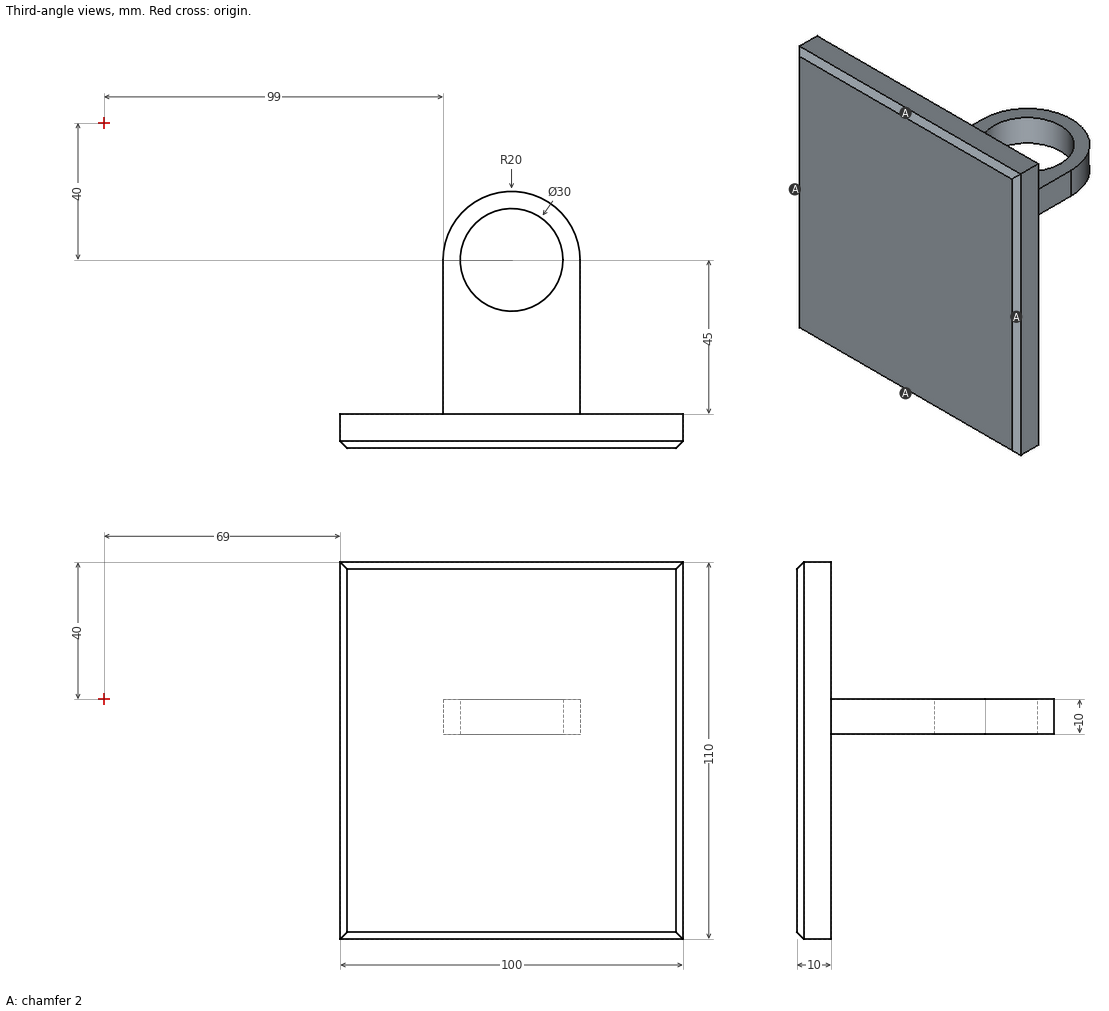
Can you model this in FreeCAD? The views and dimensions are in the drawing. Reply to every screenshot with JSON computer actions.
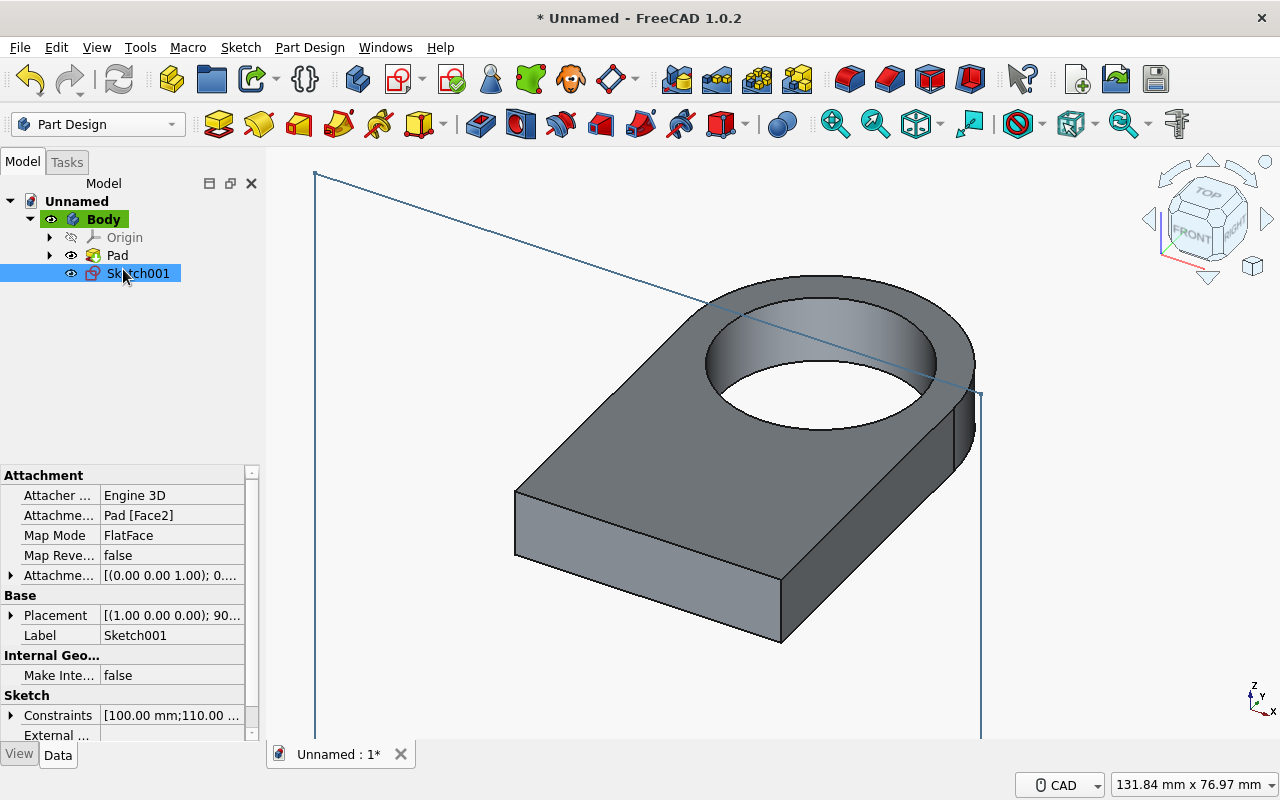
{"action": "left_click", "coordinate": [220, 124]}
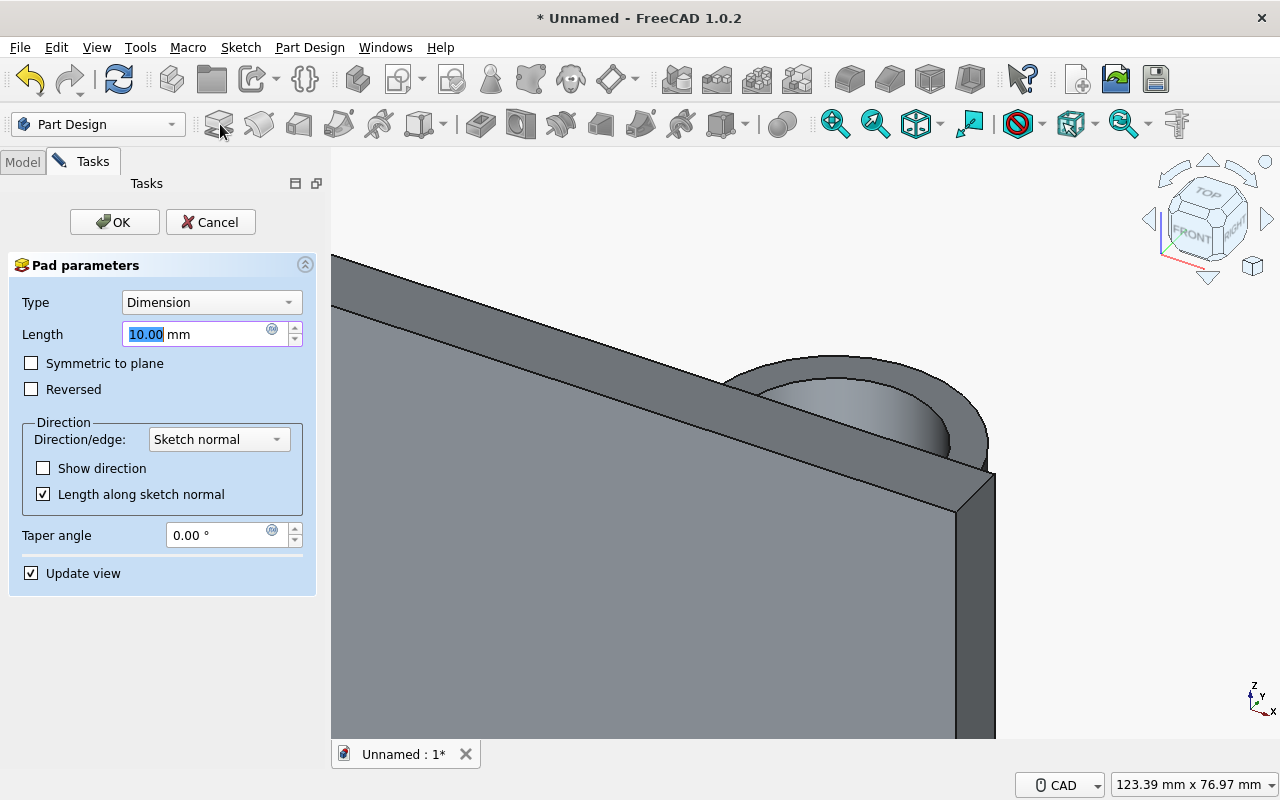
{"action": "type", "text": "10"}
{"action": "key", "text": "Tab"}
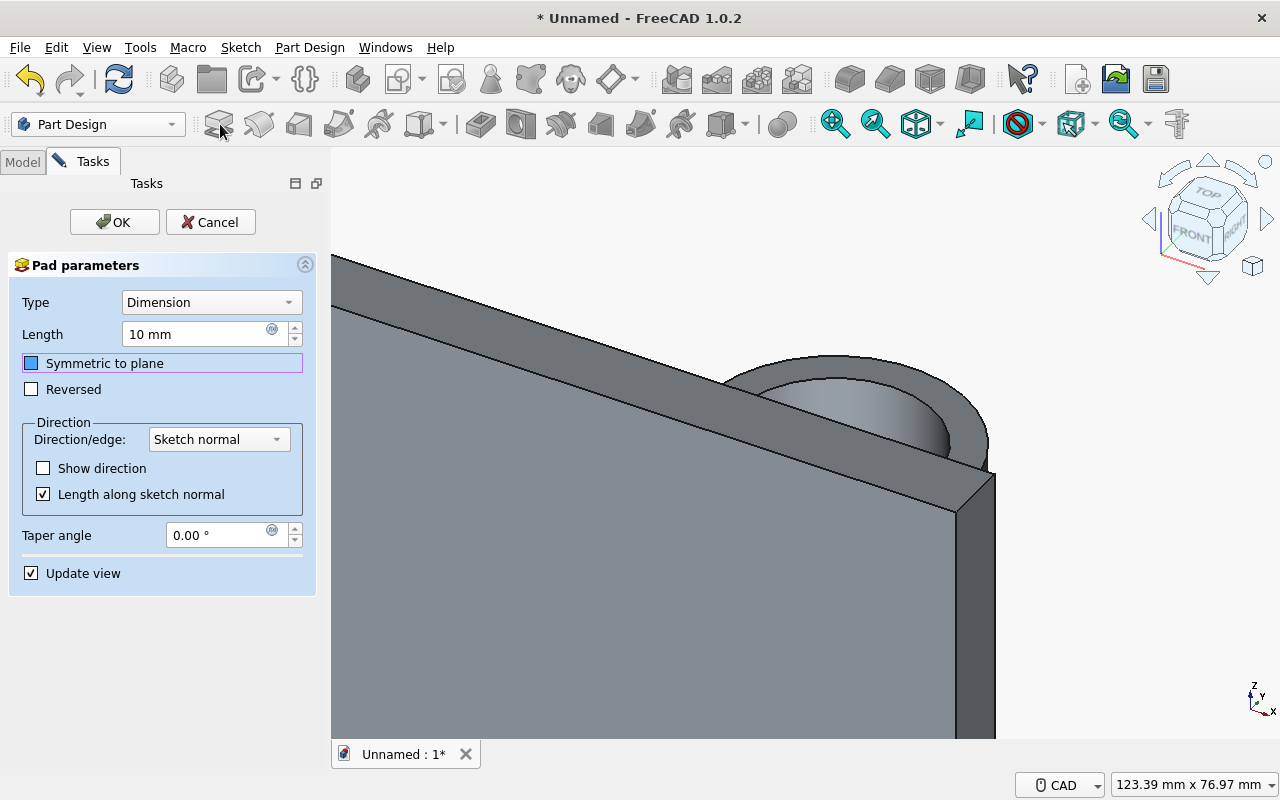
{"action": "left_click", "coordinate": [115, 222]}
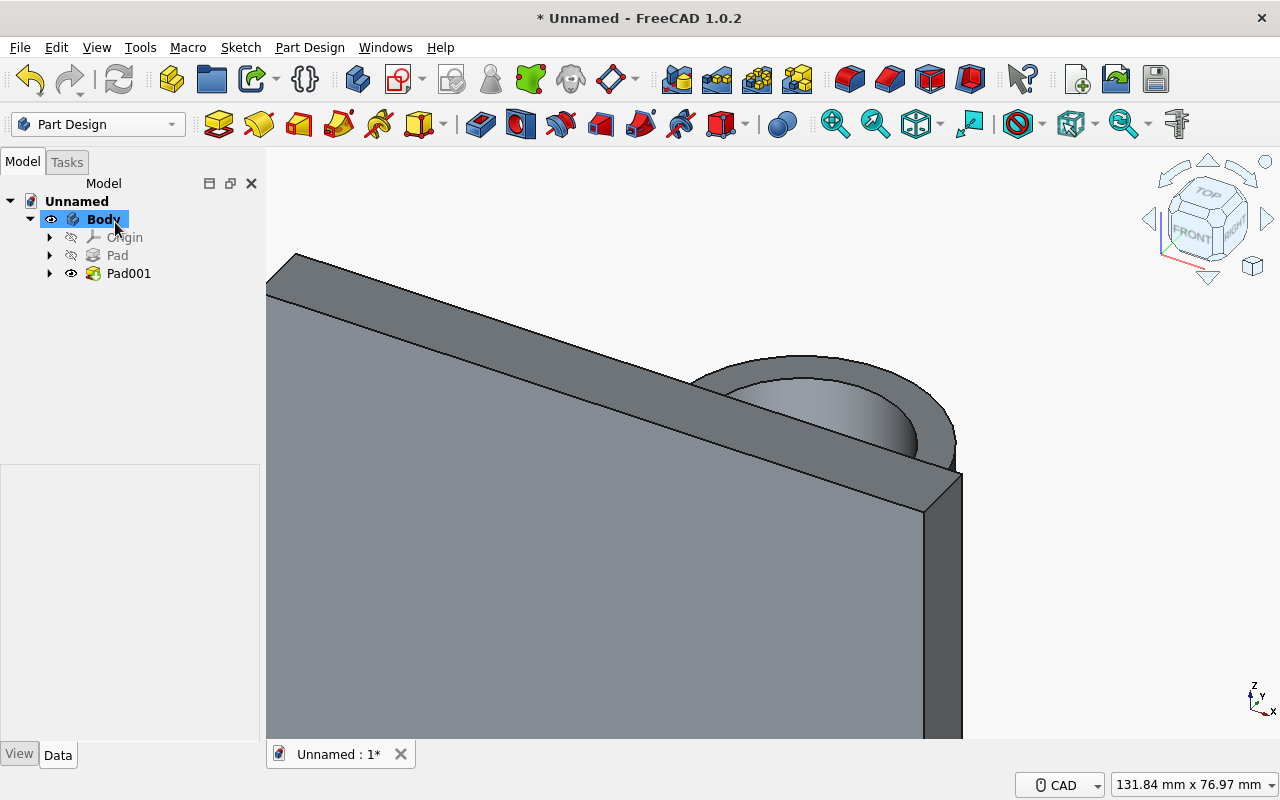
{"action": "left_click", "coordinate": [836, 124]}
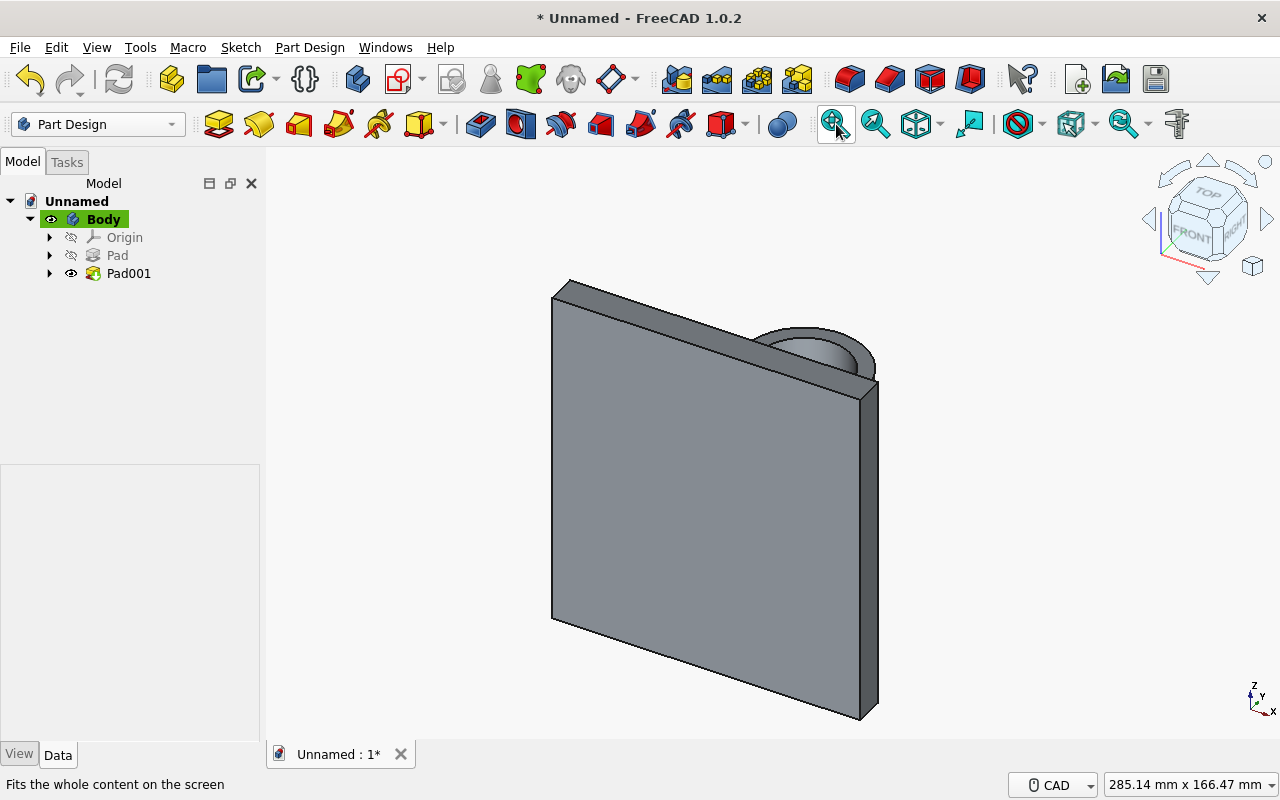
{"action": "left_click", "coordinate": [706, 508]}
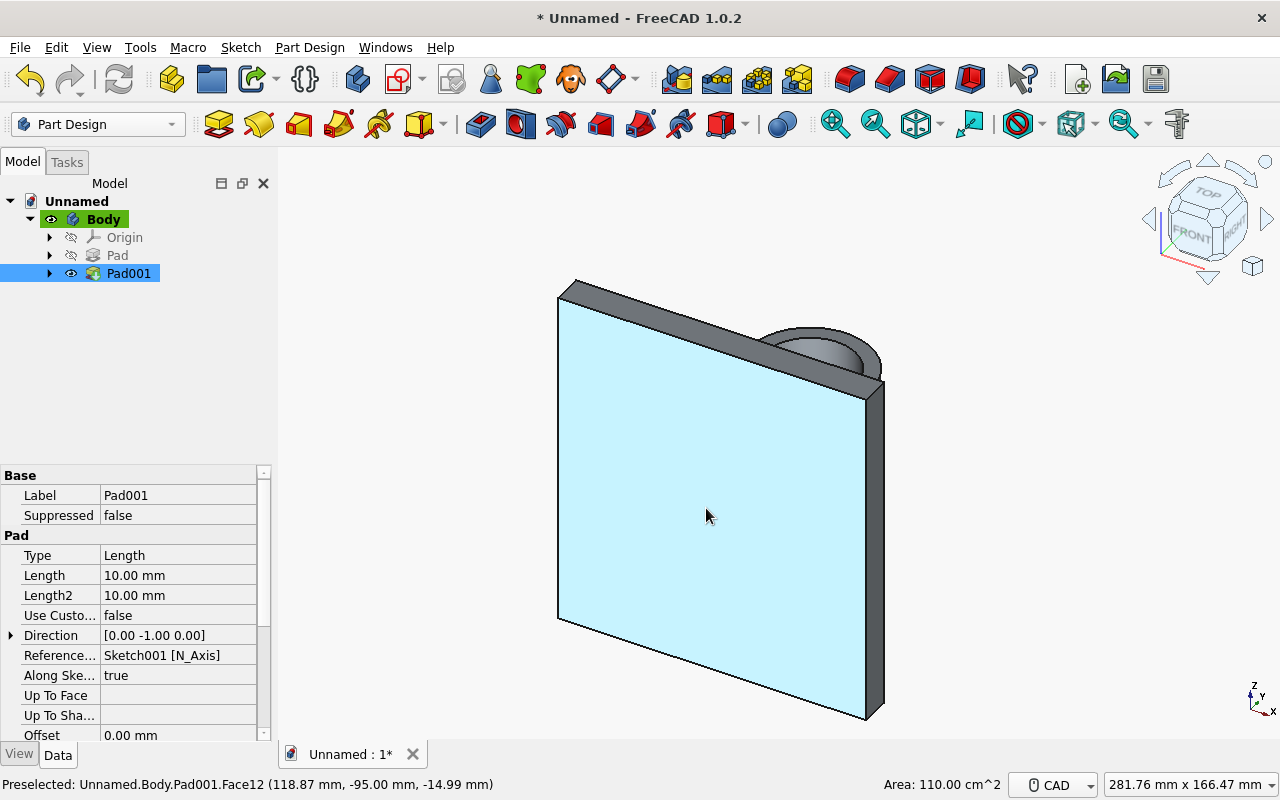
{"action": "left_click", "coordinate": [890, 80]}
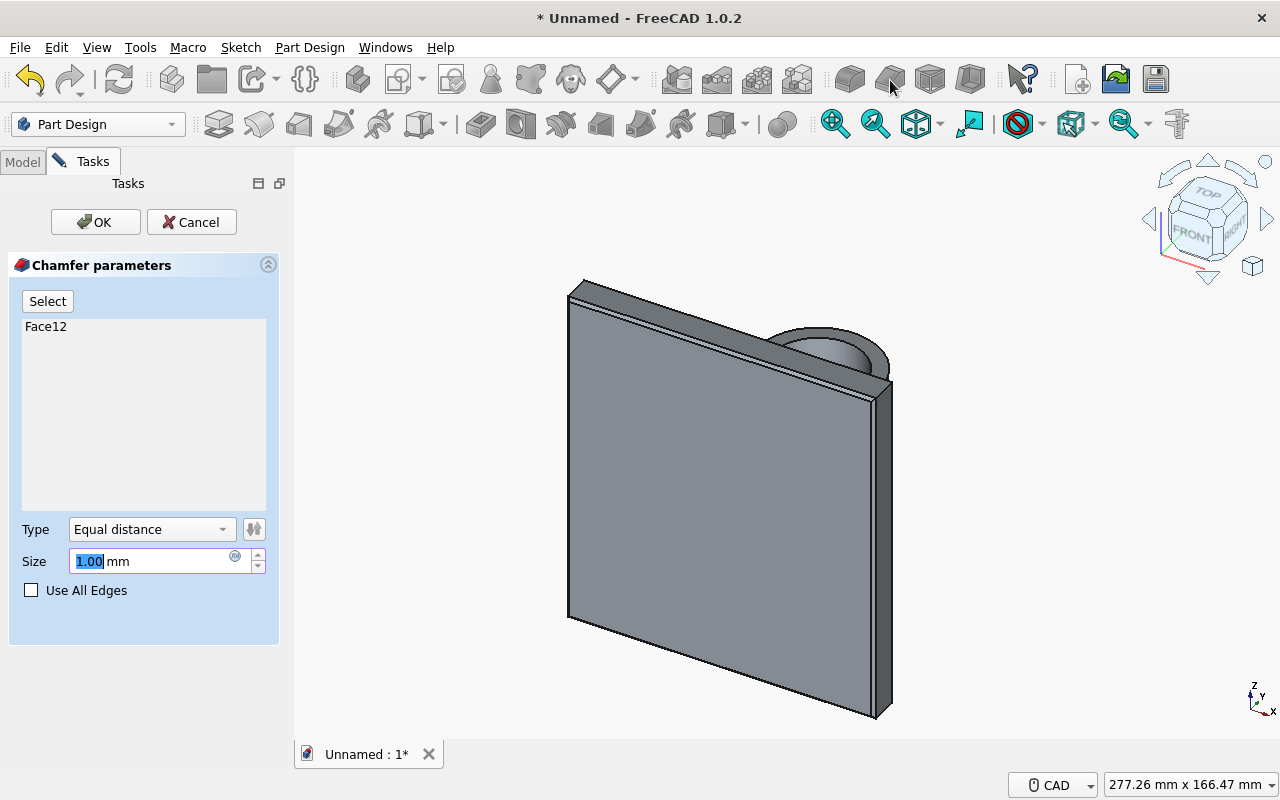
{"action": "type", "text": "2"}
{"action": "key", "text": "Tab"}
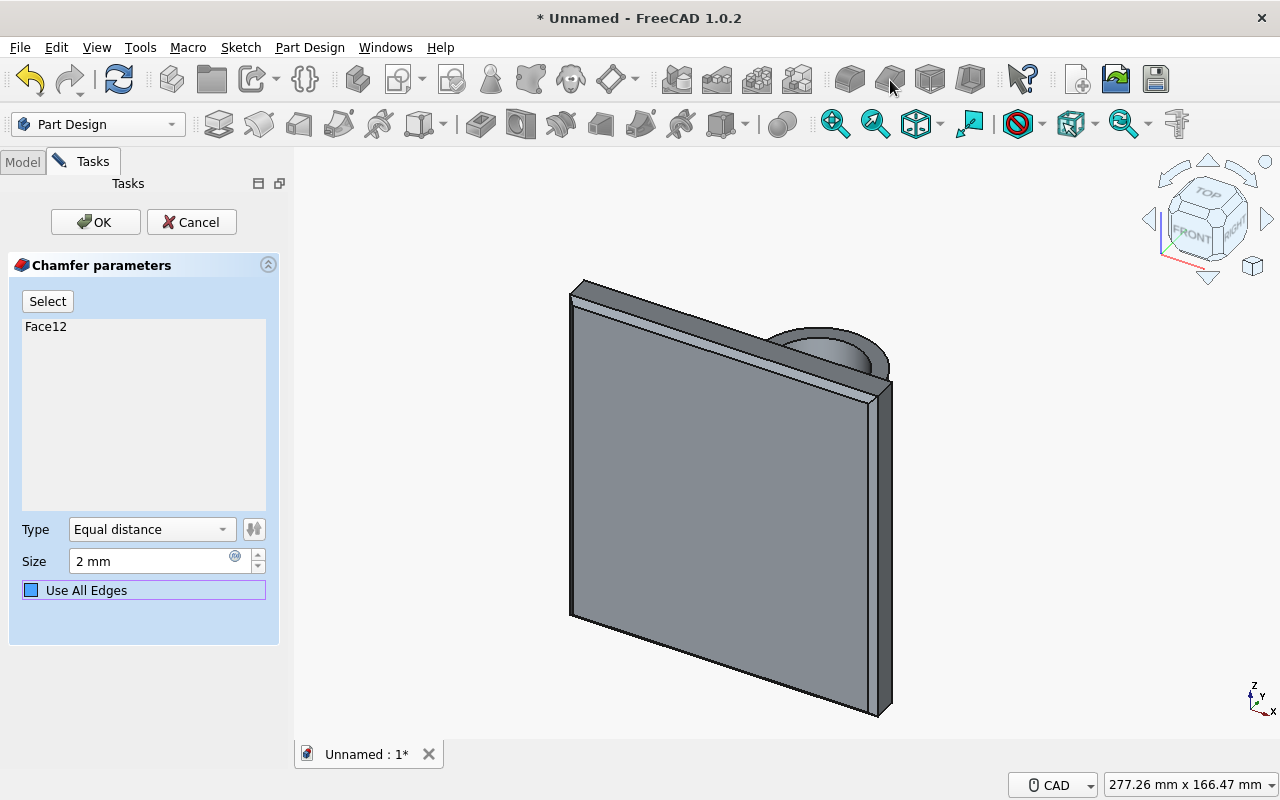
{"action": "left_click", "coordinate": [96, 222]}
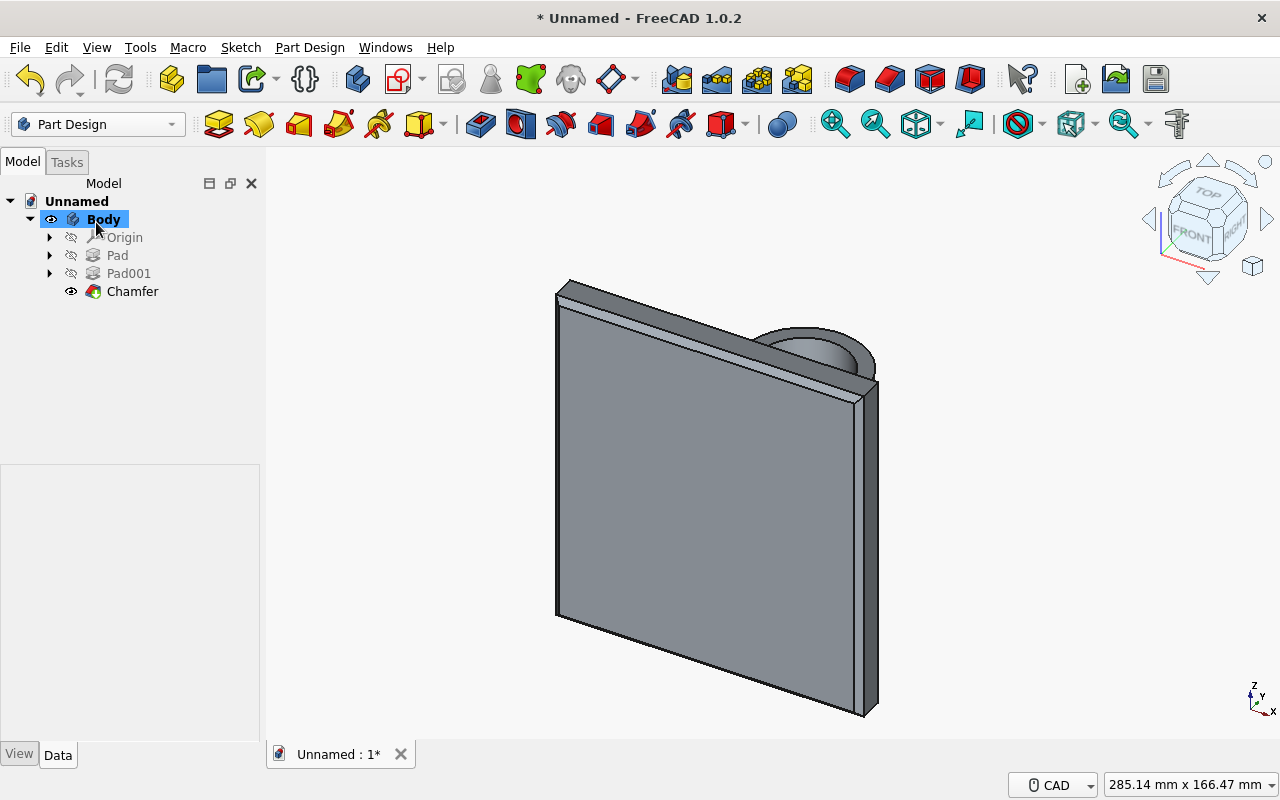
{"action": "key", "text": "0"}